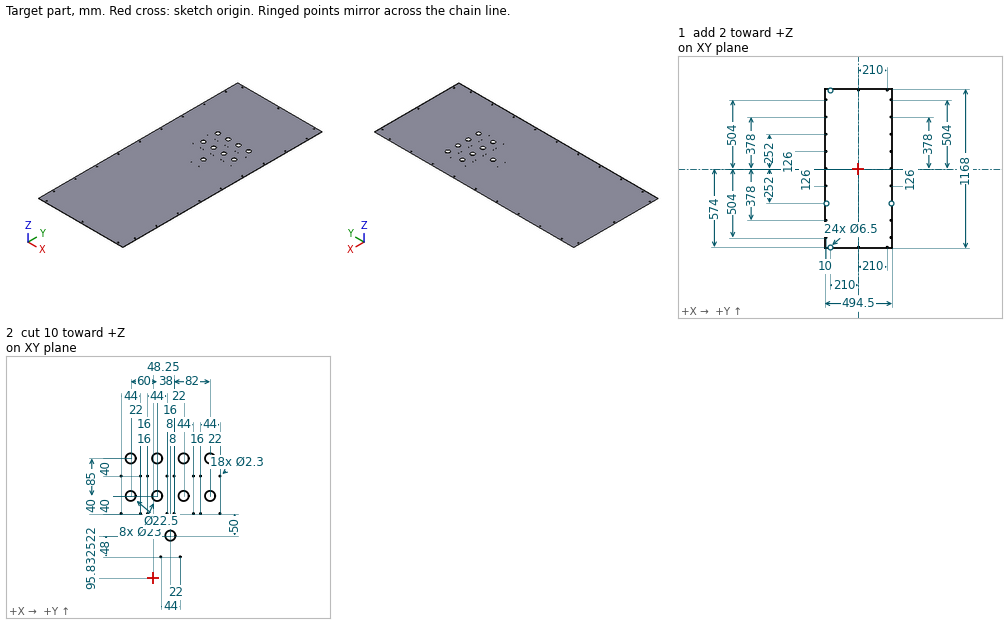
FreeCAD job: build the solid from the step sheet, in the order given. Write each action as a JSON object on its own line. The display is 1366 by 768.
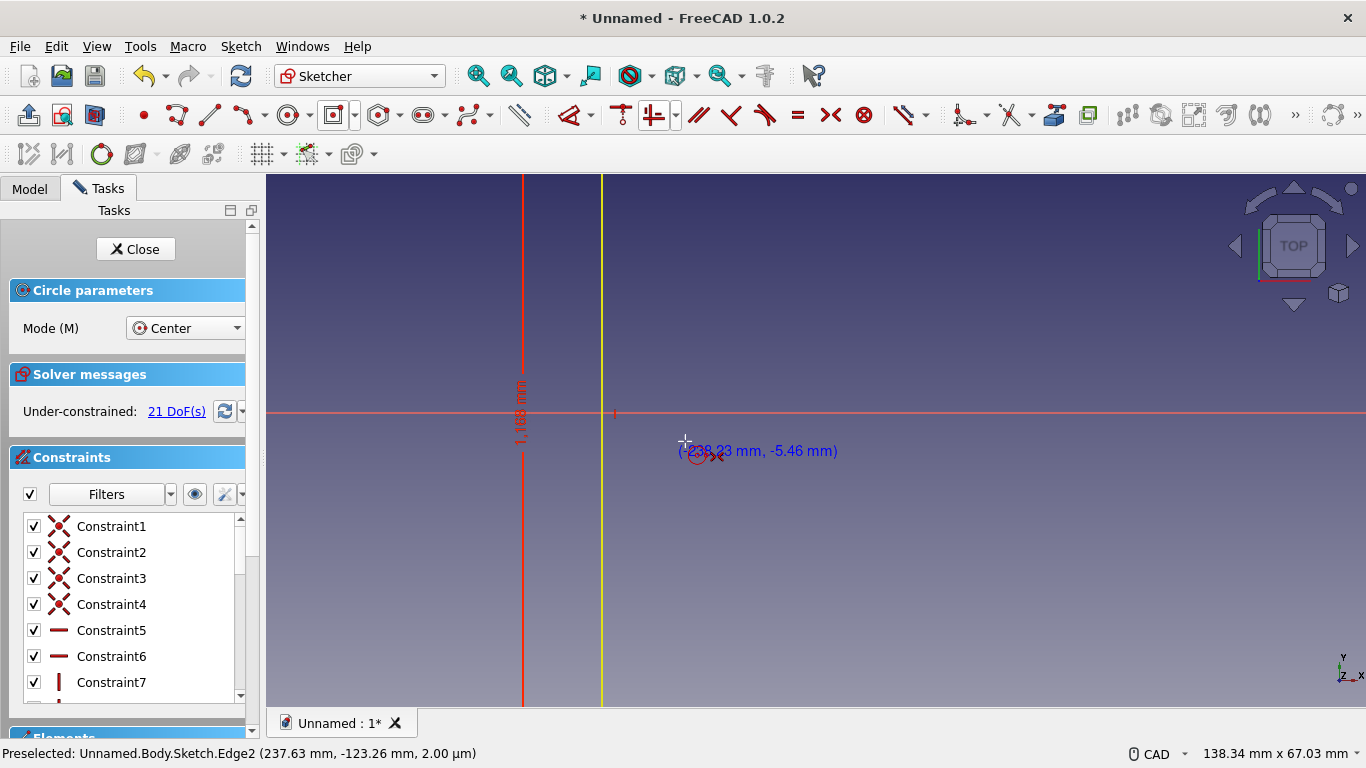
{"action": "scroll", "coordinate": [670, 442], "scroll_direction": "down", "scroll_amount": 16}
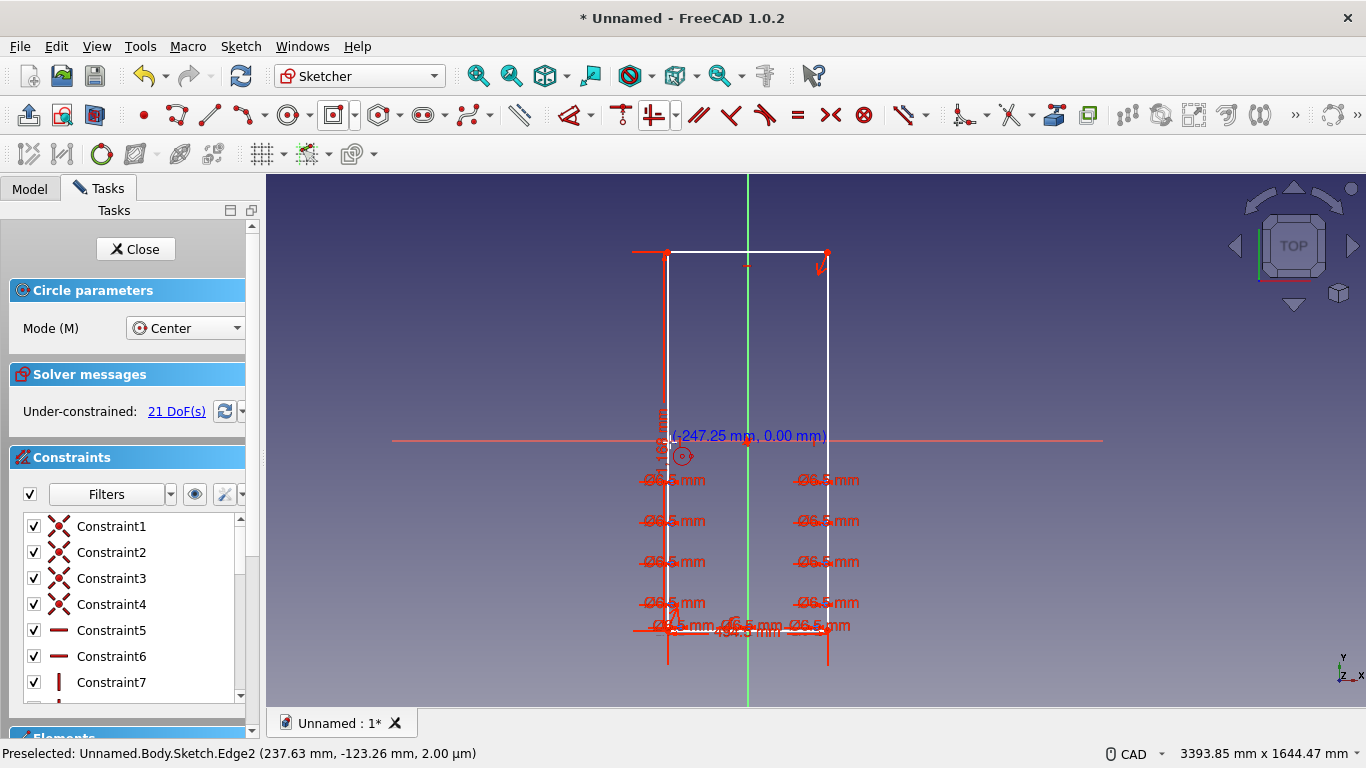
{"action": "scroll", "coordinate": [671, 441], "scroll_direction": "up", "scroll_amount": 8}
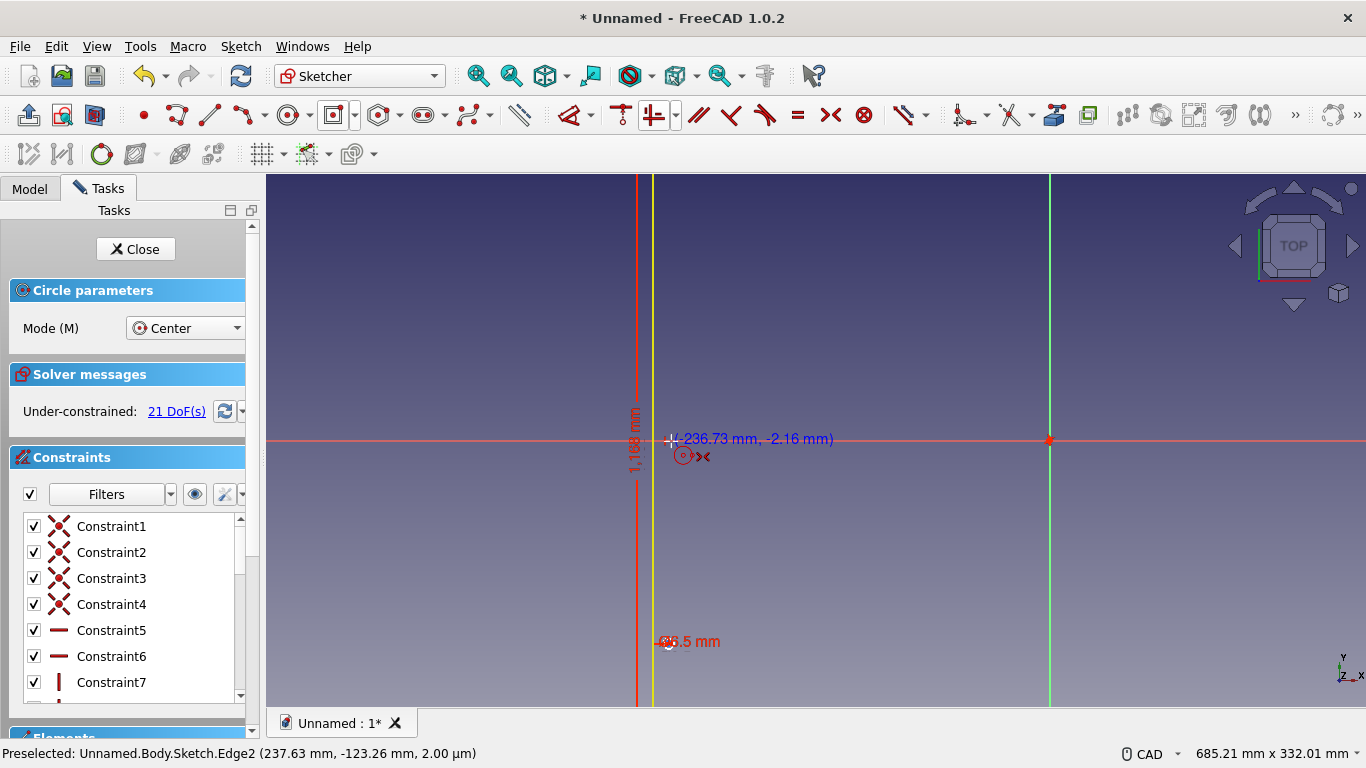
{"action": "left_click", "coordinate": [669, 441]}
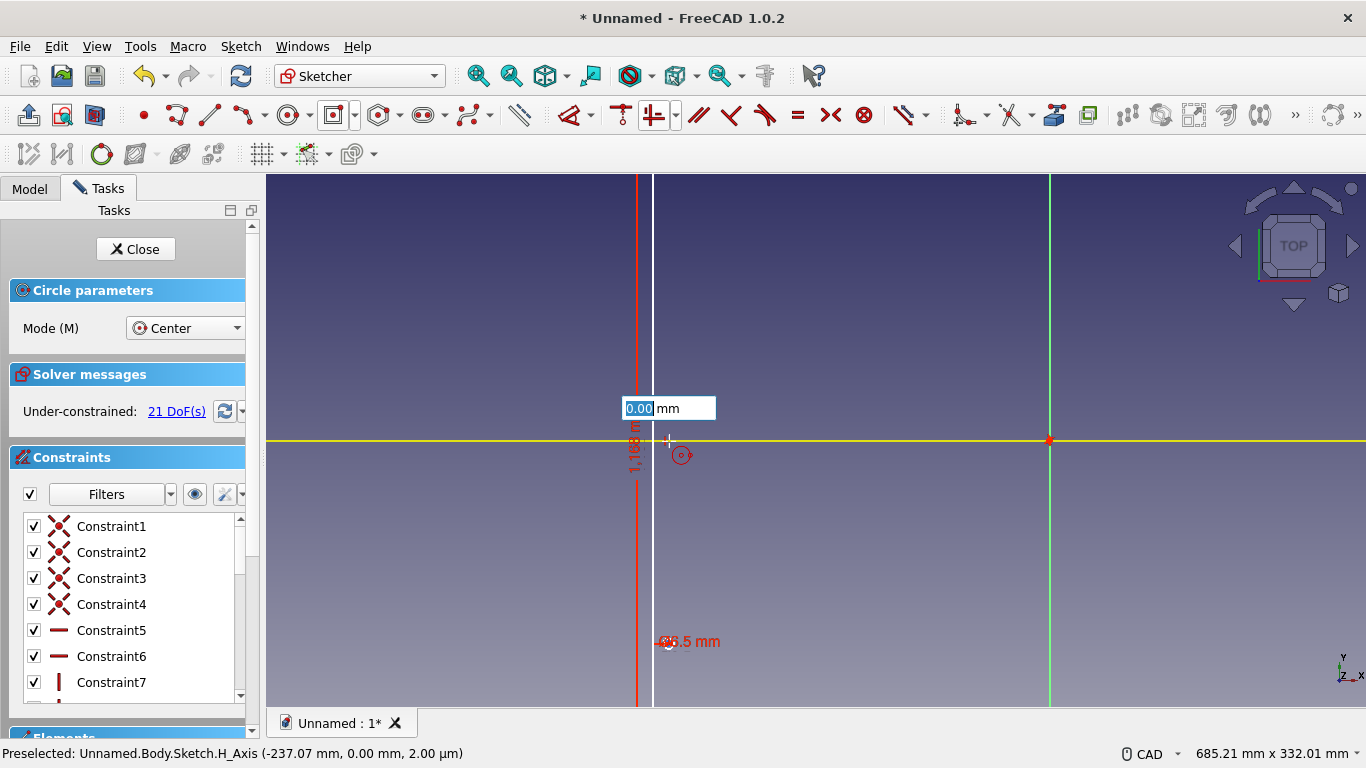
{"action": "scroll", "coordinate": [667, 445], "scroll_direction": "up", "scroll_amount": 6}
{"action": "mouse_move", "coordinate": [666, 445]}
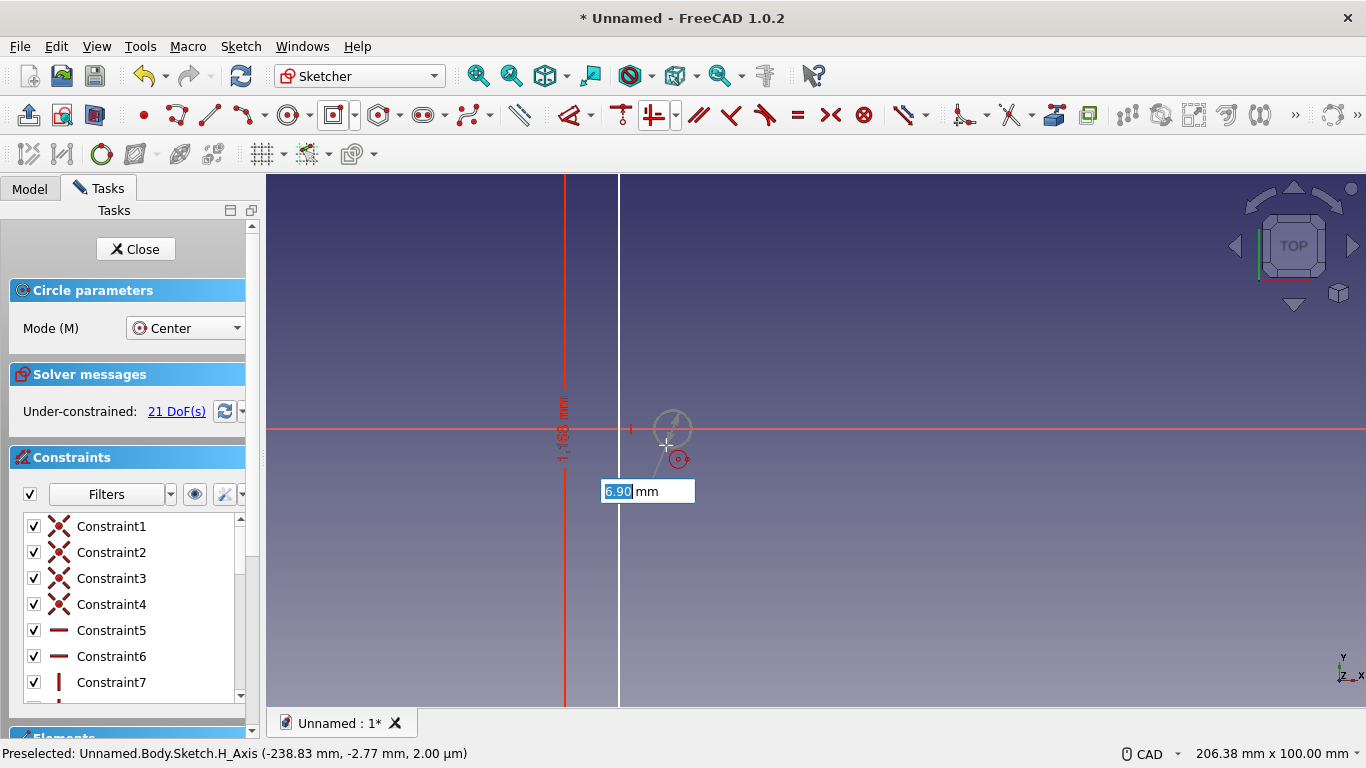
{"action": "type", "text": "6.5"}
{"action": "key", "text": "Return"}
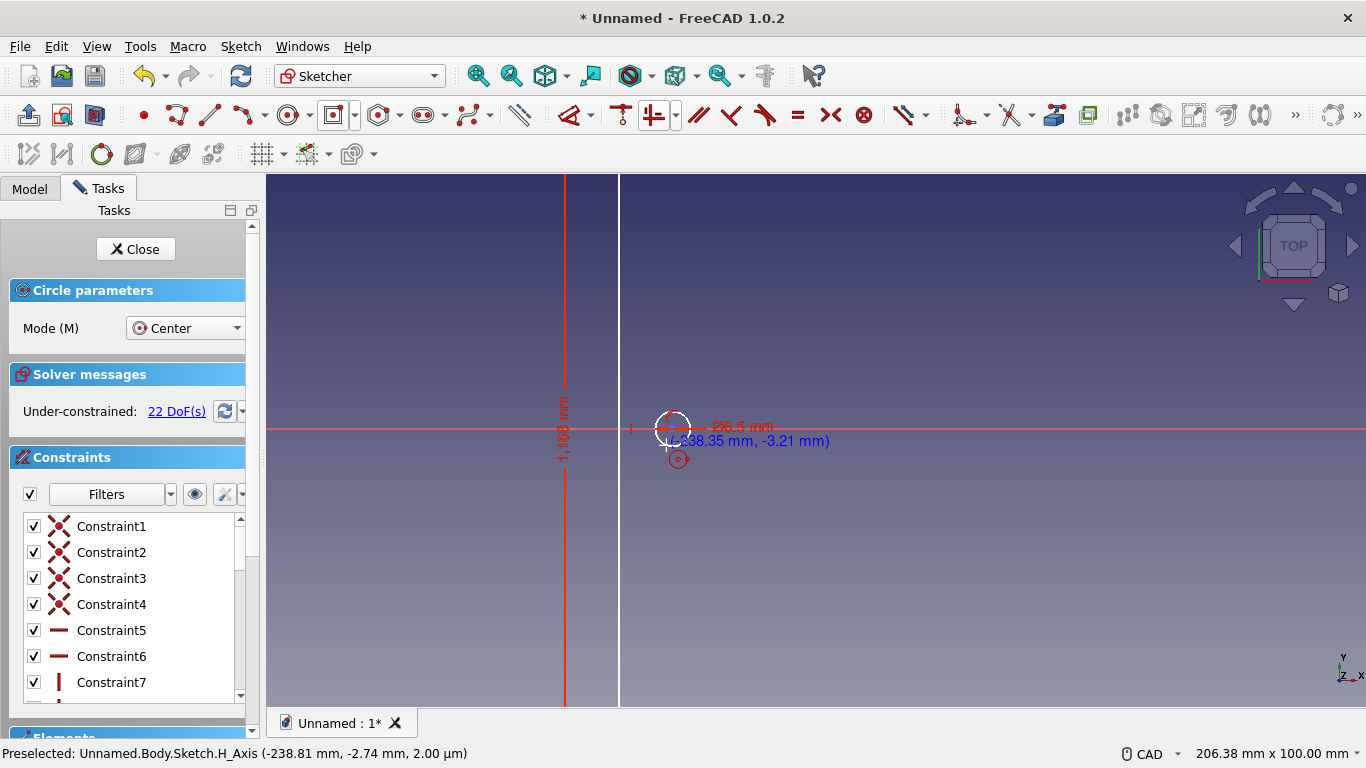
{"action": "scroll", "coordinate": [685, 441], "scroll_direction": "down", "scroll_amount": 15}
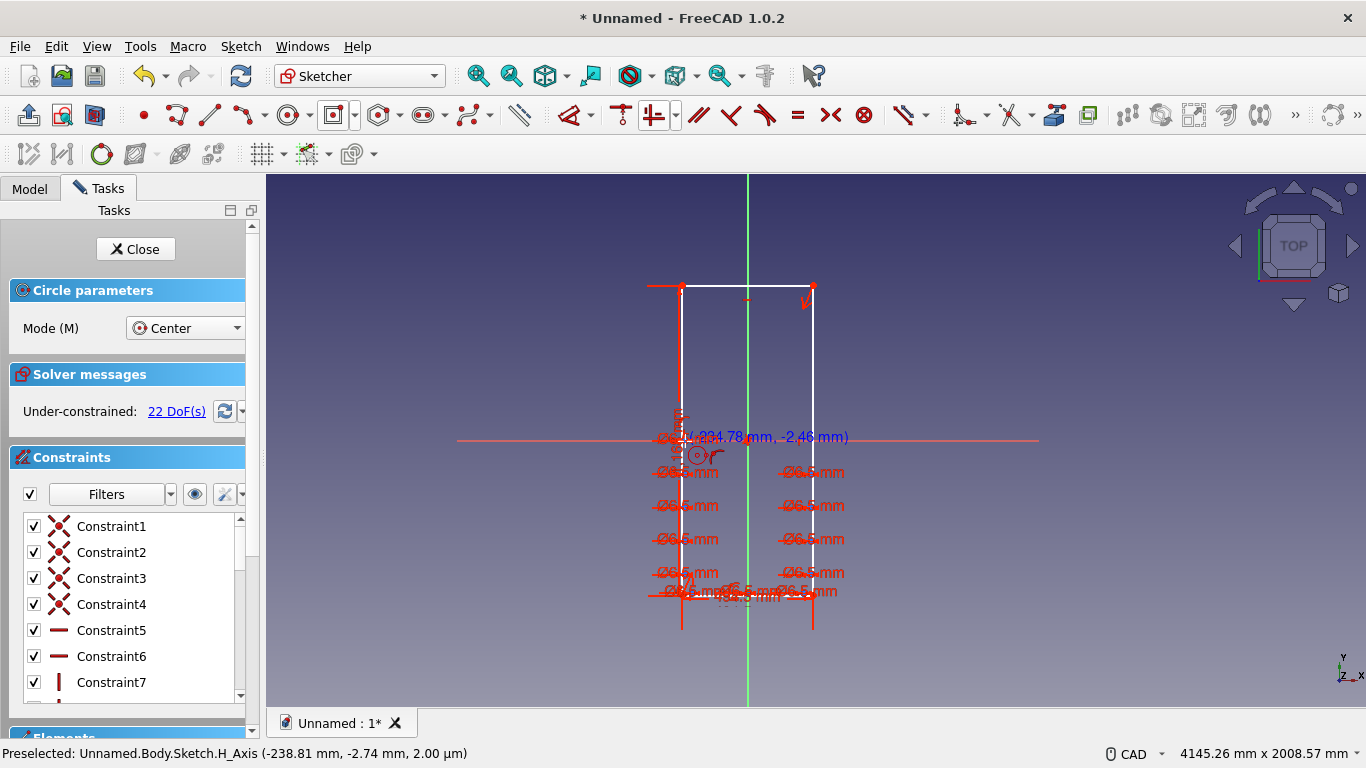
{"action": "scroll", "coordinate": [685, 407], "scroll_direction": "up", "scroll_amount": 17}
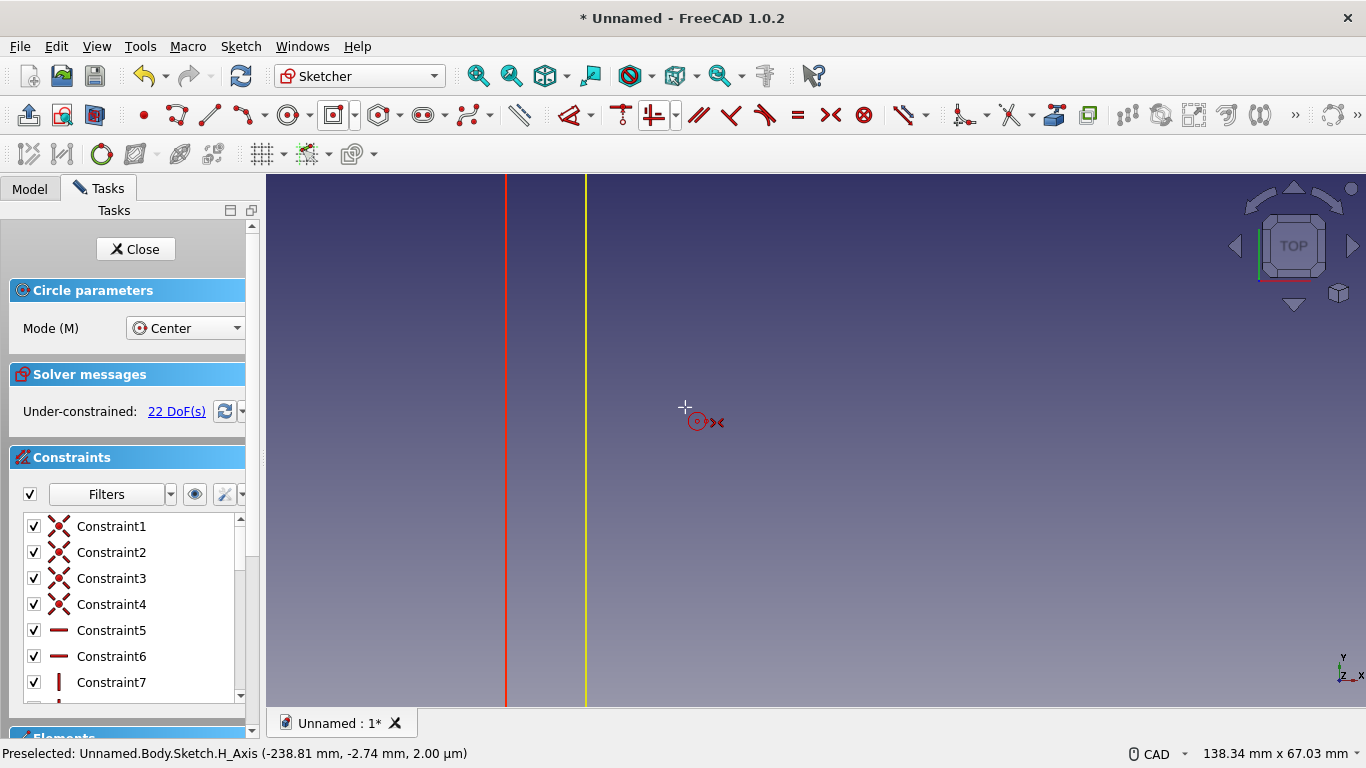
{"action": "scroll", "coordinate": [671, 399], "scroll_direction": "down", "scroll_amount": 16}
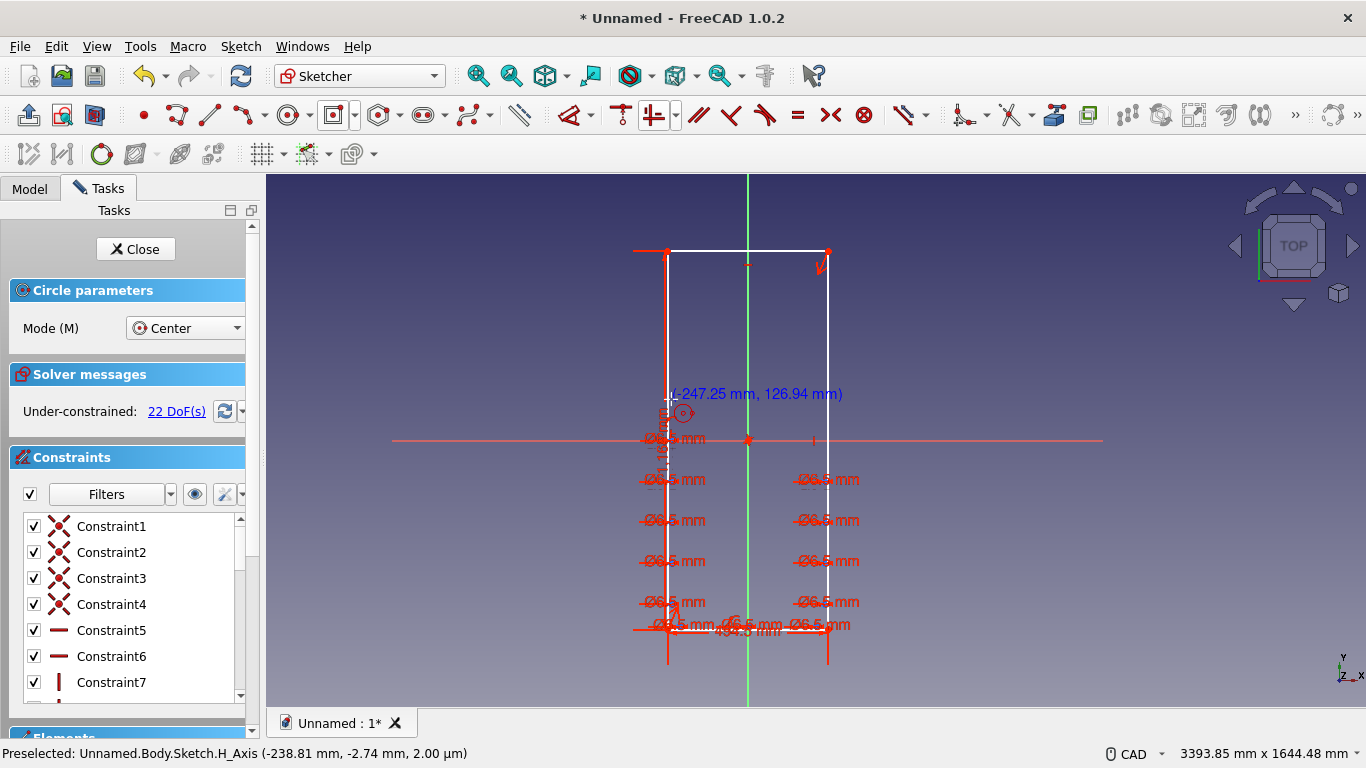
{"action": "scroll", "coordinate": [671, 400], "scroll_direction": "up", "scroll_amount": 8}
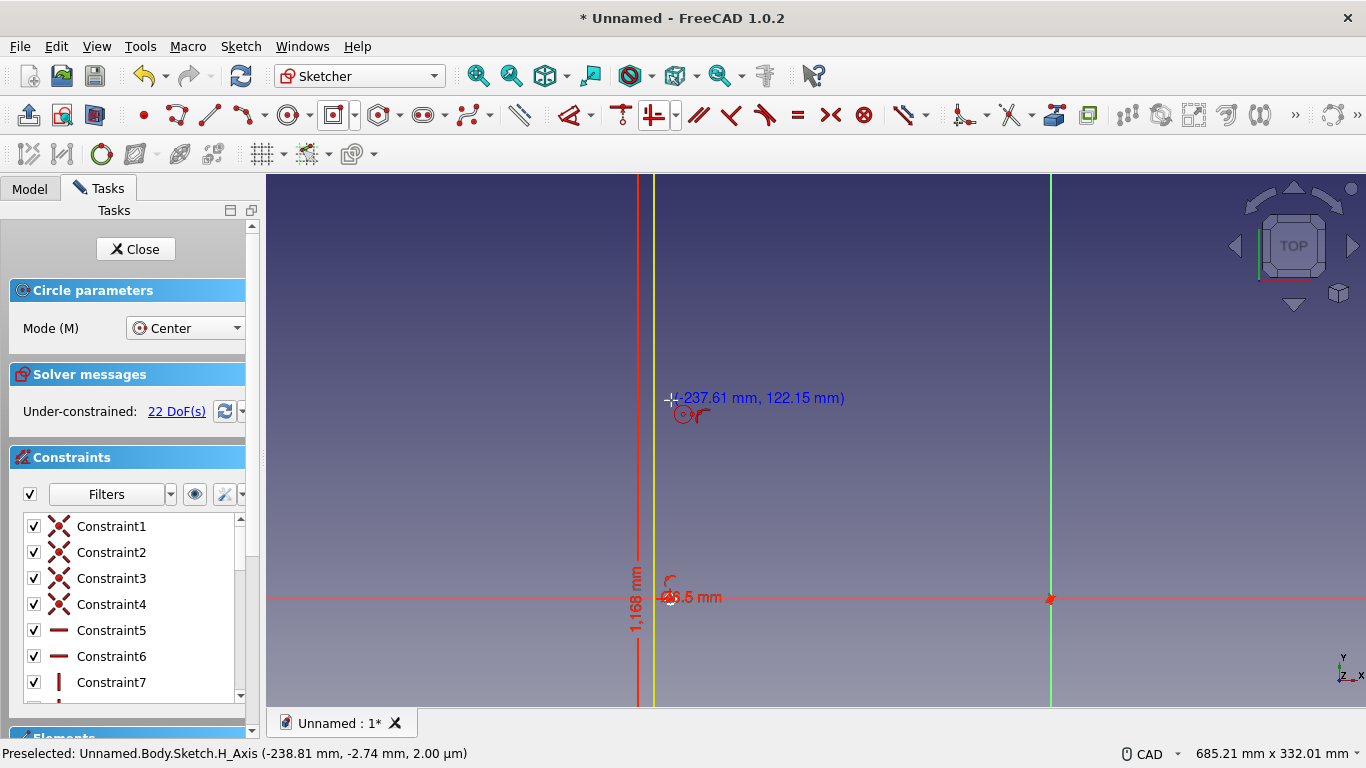
{"action": "left_click", "coordinate": [670, 397]}
{"action": "mouse_move", "coordinate": [674, 393]}